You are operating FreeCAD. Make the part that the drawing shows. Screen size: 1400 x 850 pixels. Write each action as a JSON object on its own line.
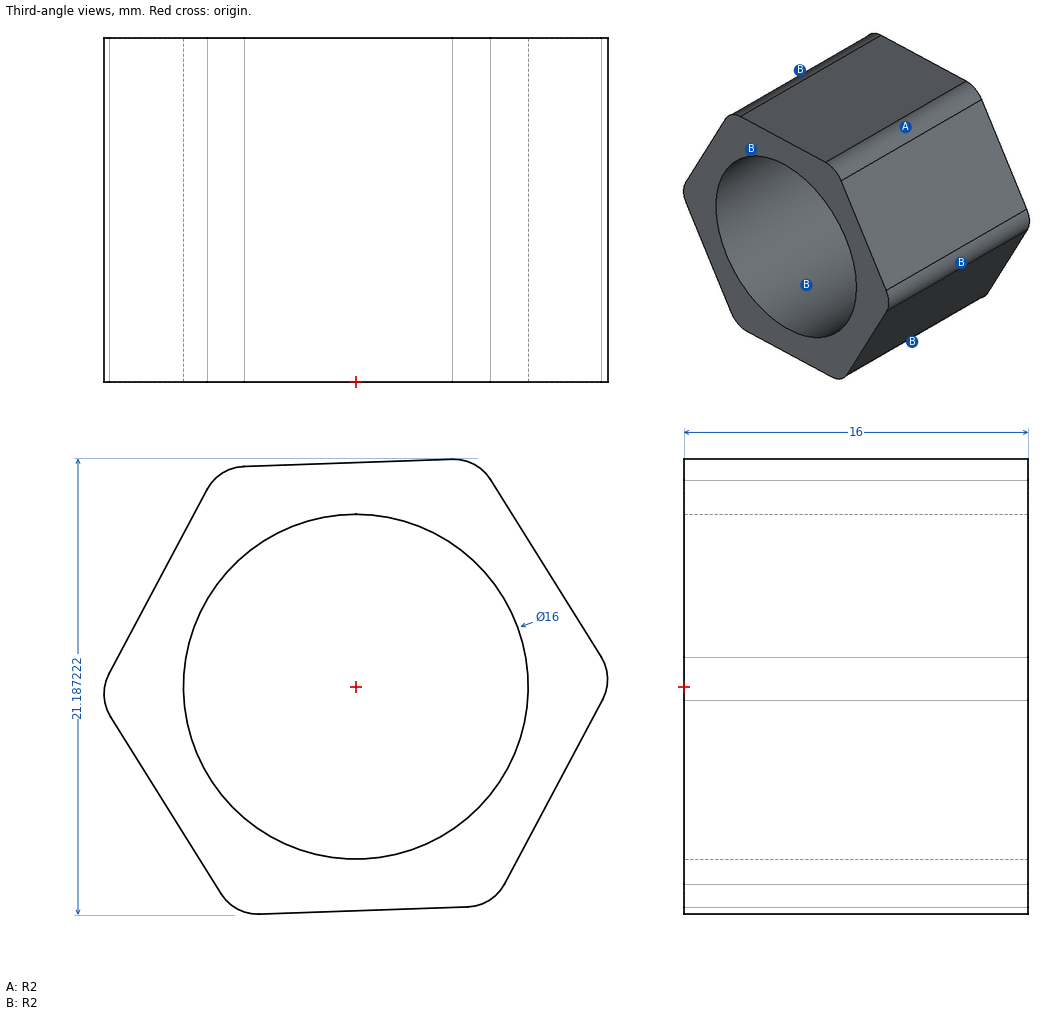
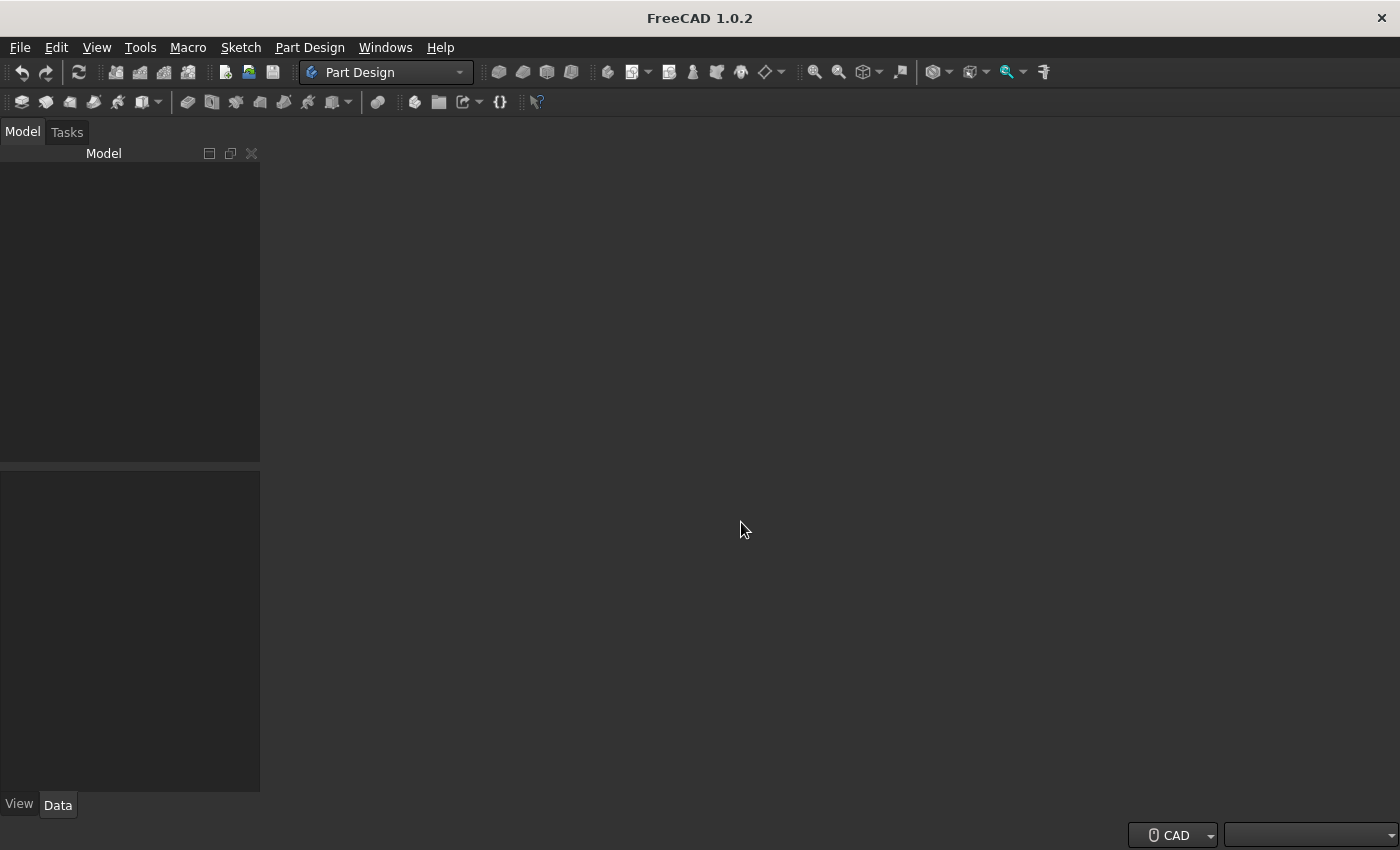
{"action": "left_click", "coordinate": [226, 72]}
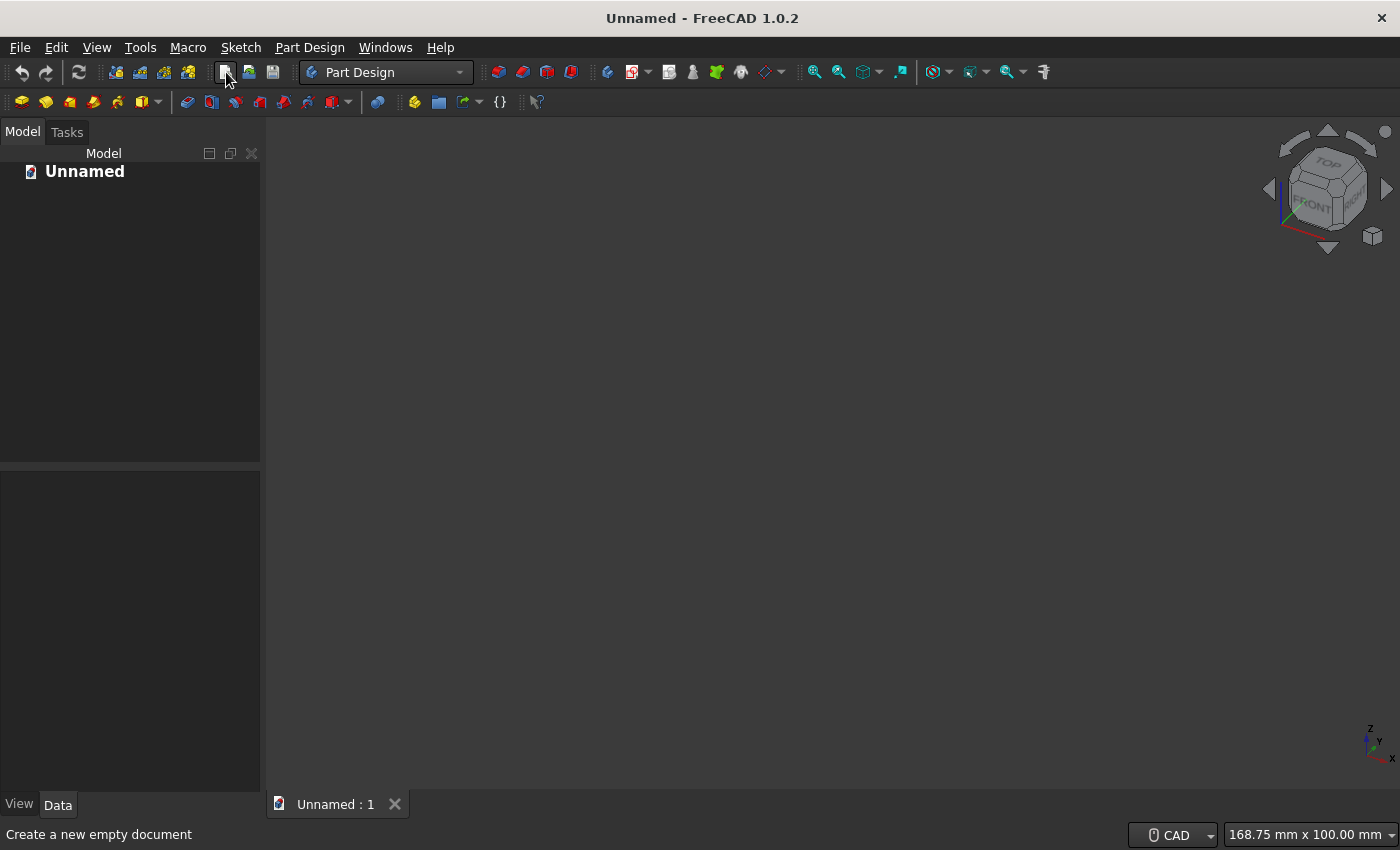
{"action": "left_click", "coordinate": [632, 72]}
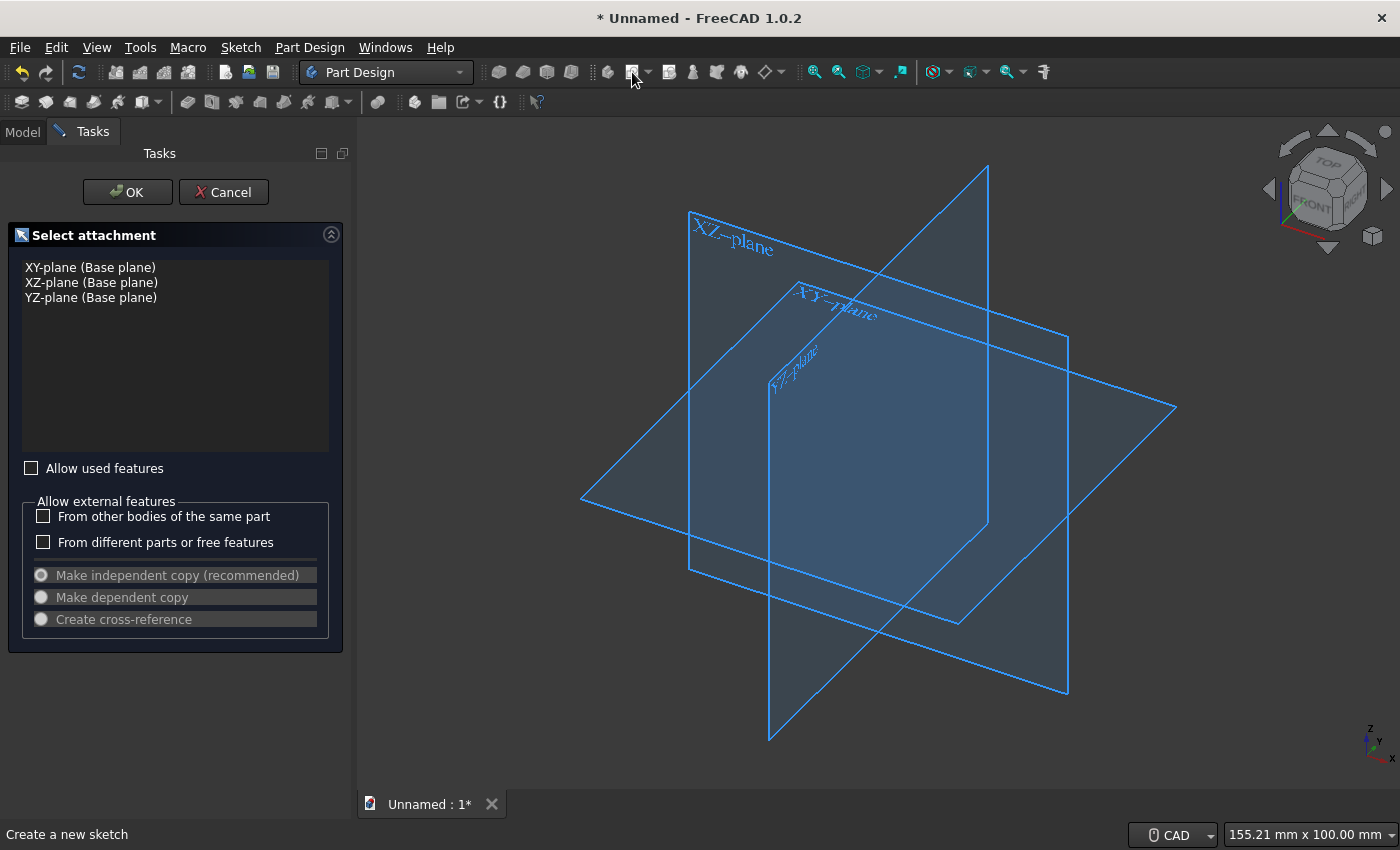
{"action": "left_click", "coordinate": [82, 282]}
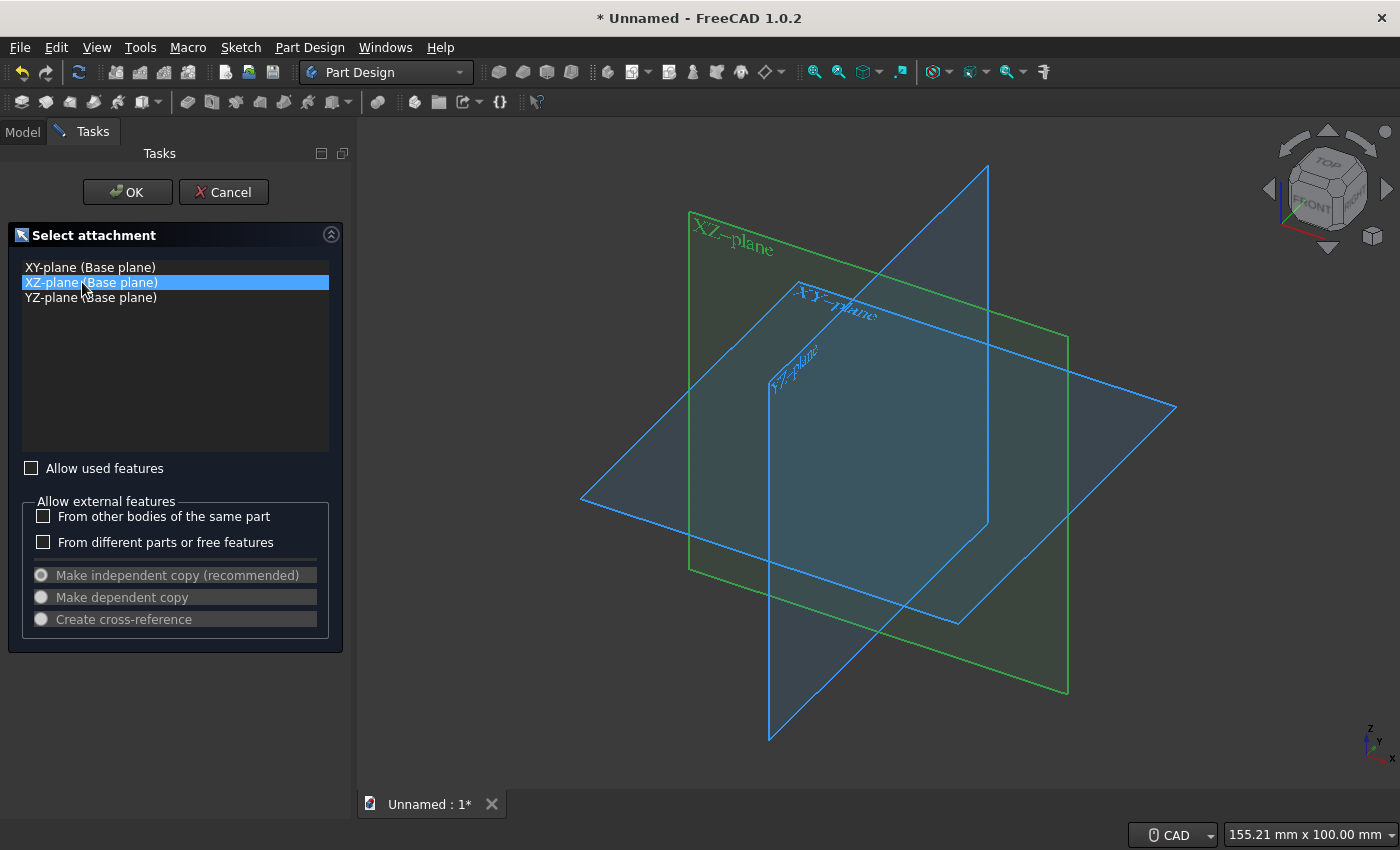
{"action": "left_click", "coordinate": [128, 192]}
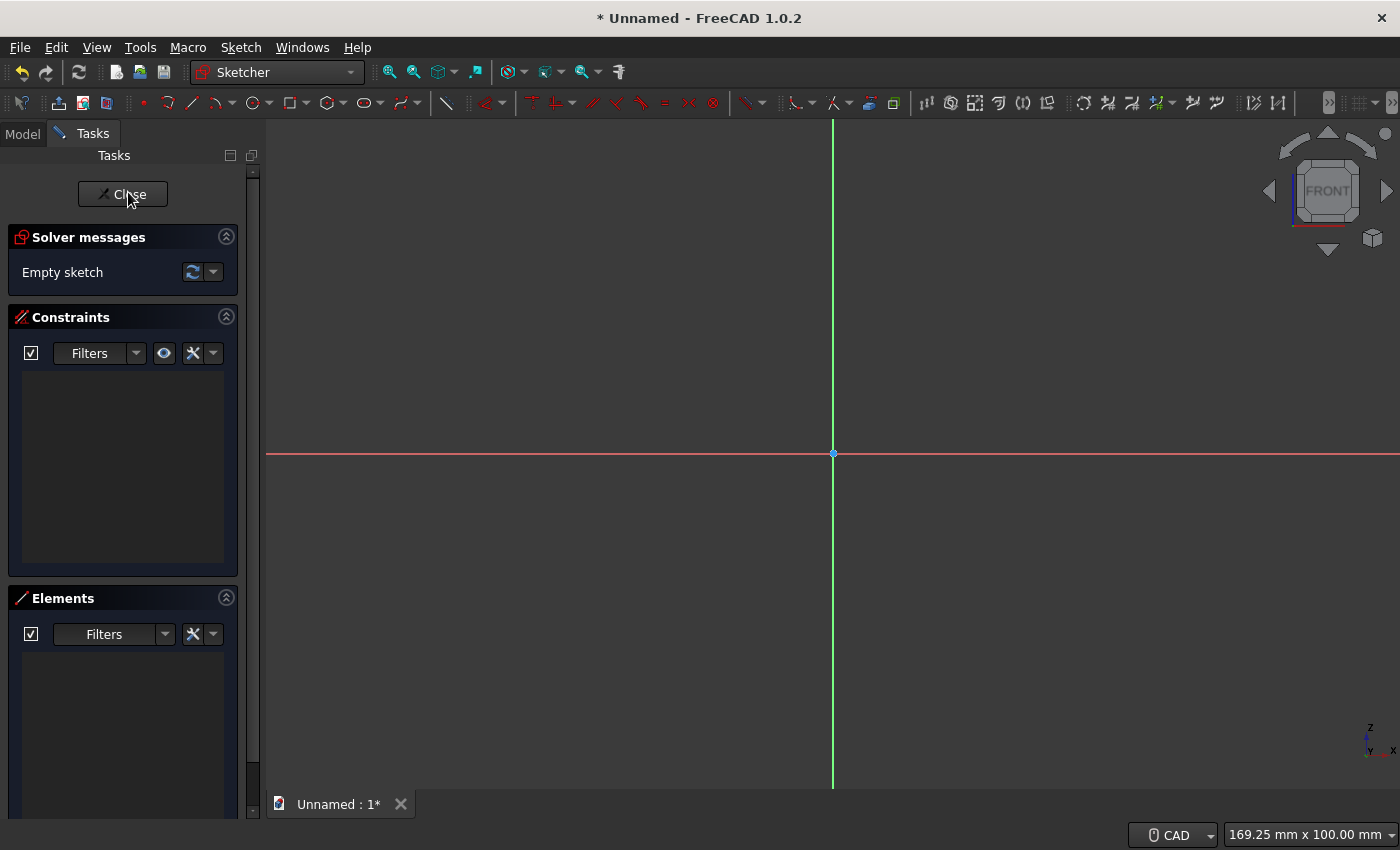
{"action": "scroll", "coordinate": [863, 454], "scroll_direction": "up", "scroll_amount": 6}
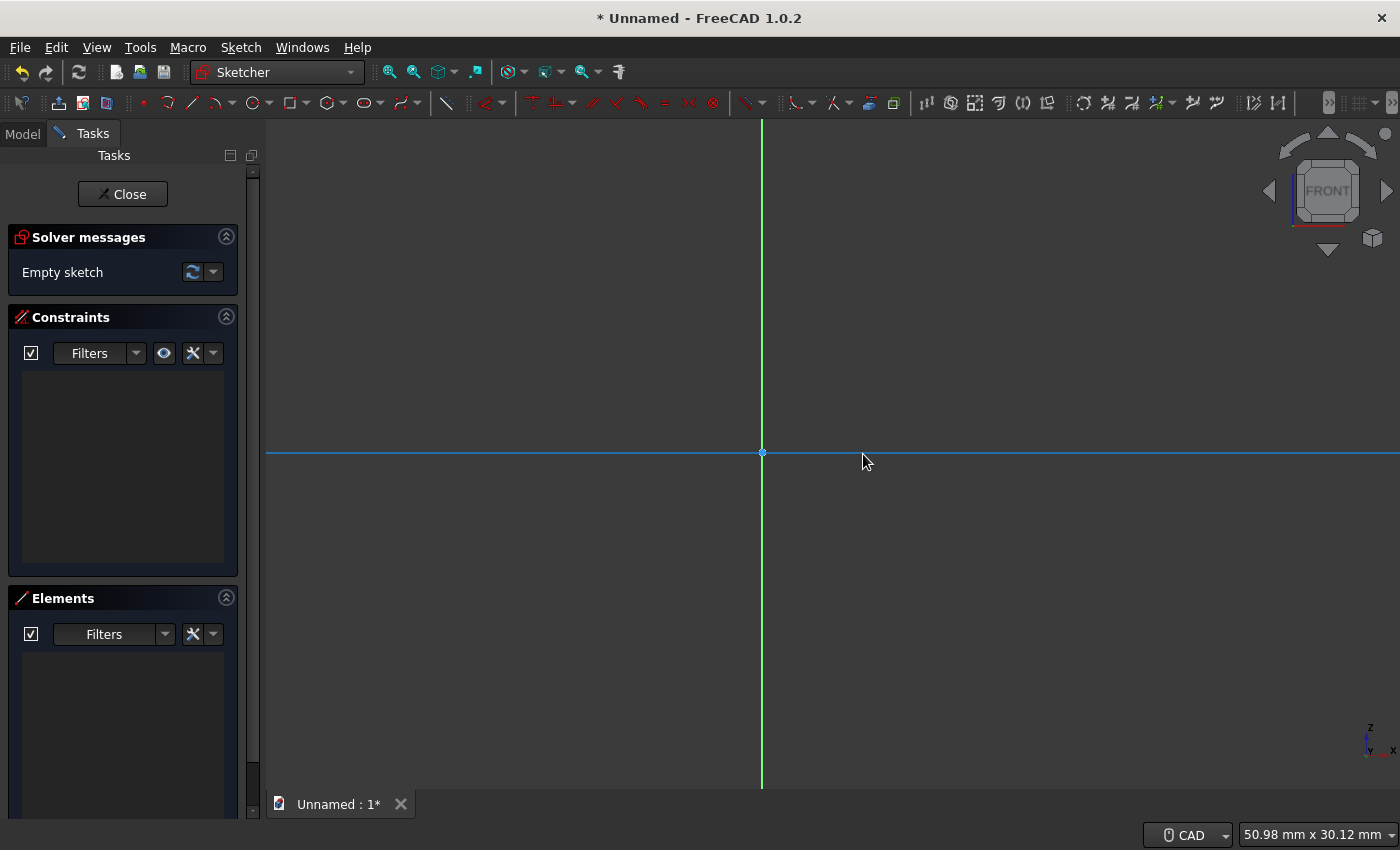
{"action": "left_click", "coordinate": [328, 104]}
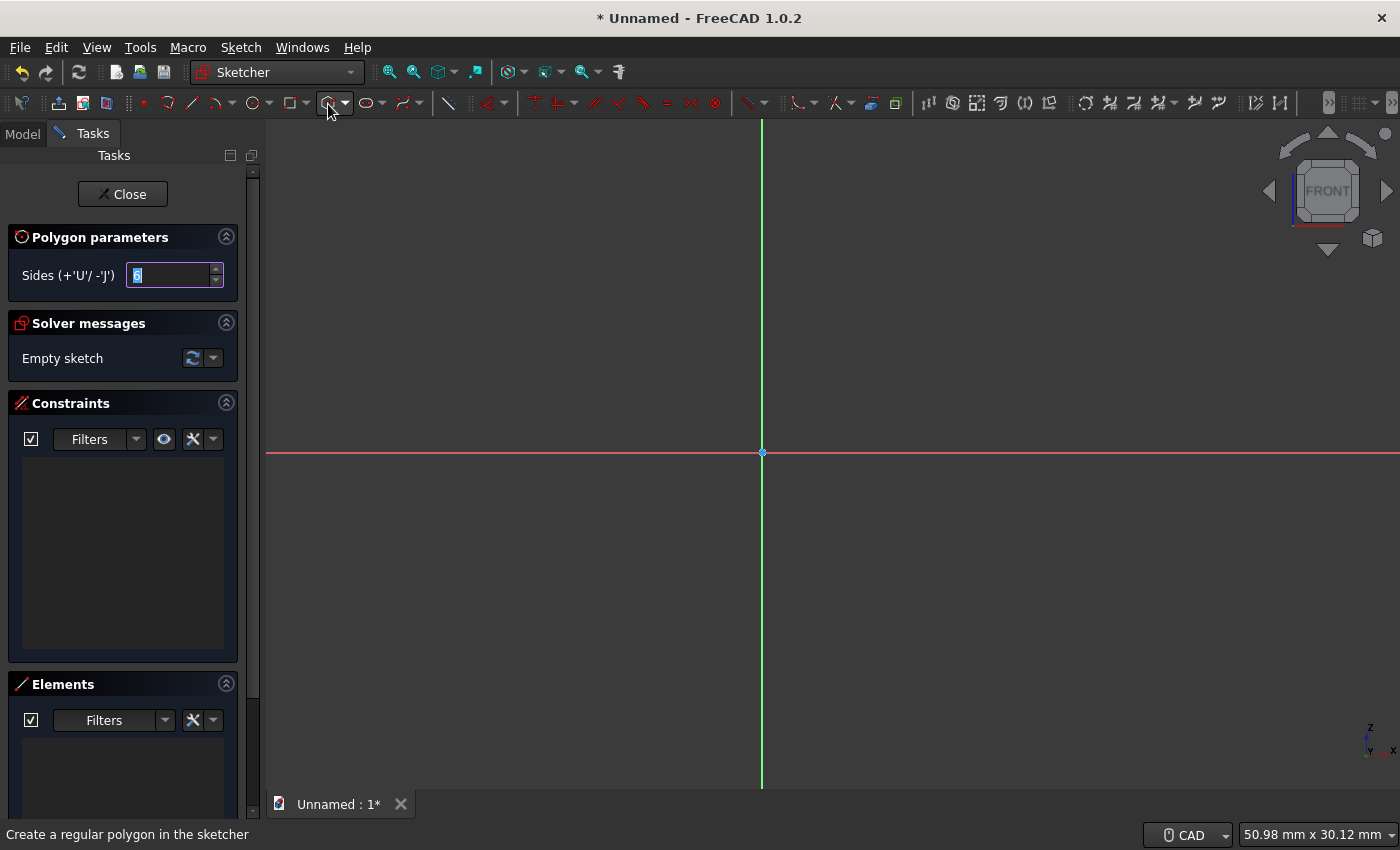
{"action": "left_click", "coordinate": [762, 453]}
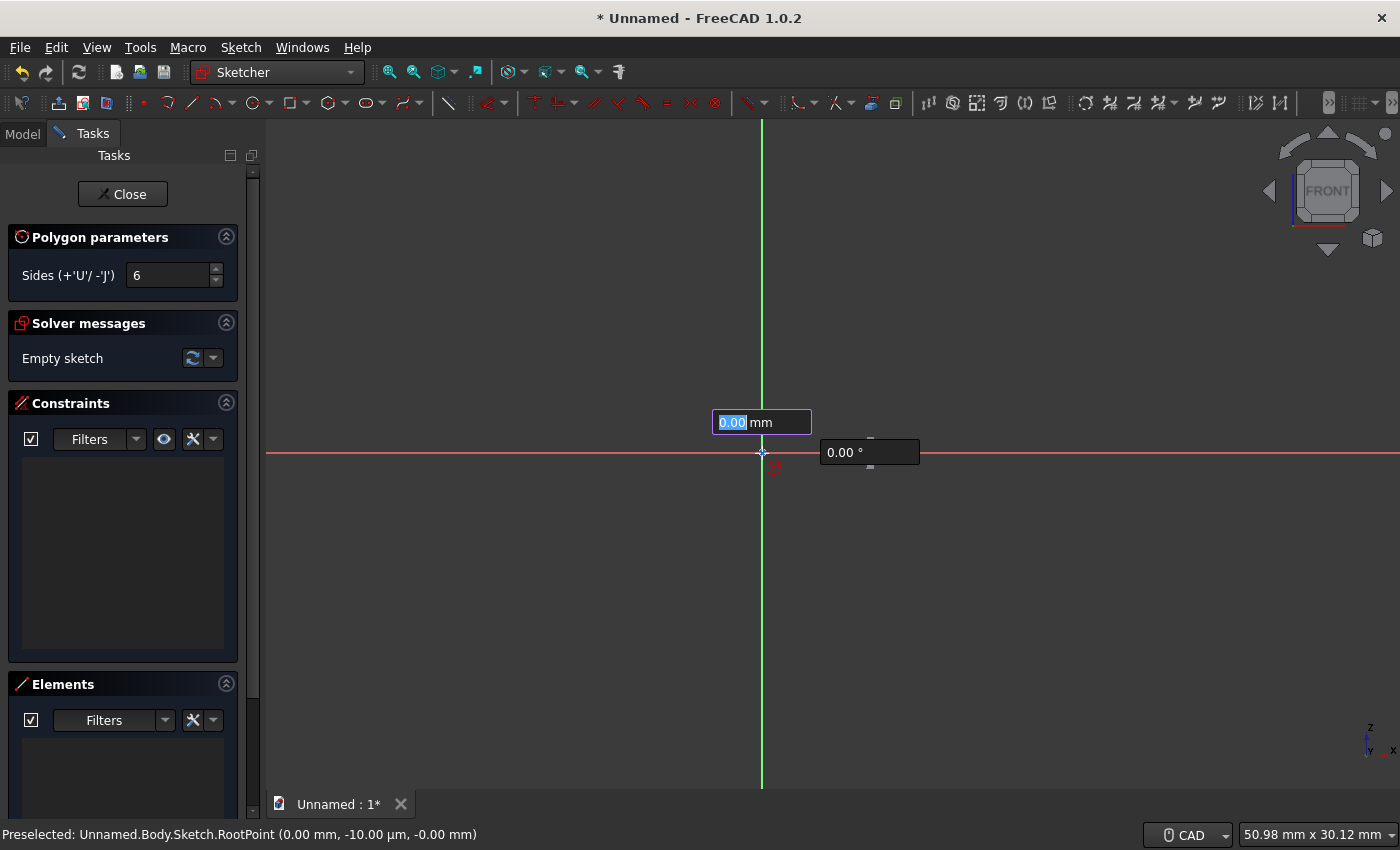
{"action": "left_click", "coordinate": [904, 679]}
{"action": "right_click", "coordinate": [904, 679]}